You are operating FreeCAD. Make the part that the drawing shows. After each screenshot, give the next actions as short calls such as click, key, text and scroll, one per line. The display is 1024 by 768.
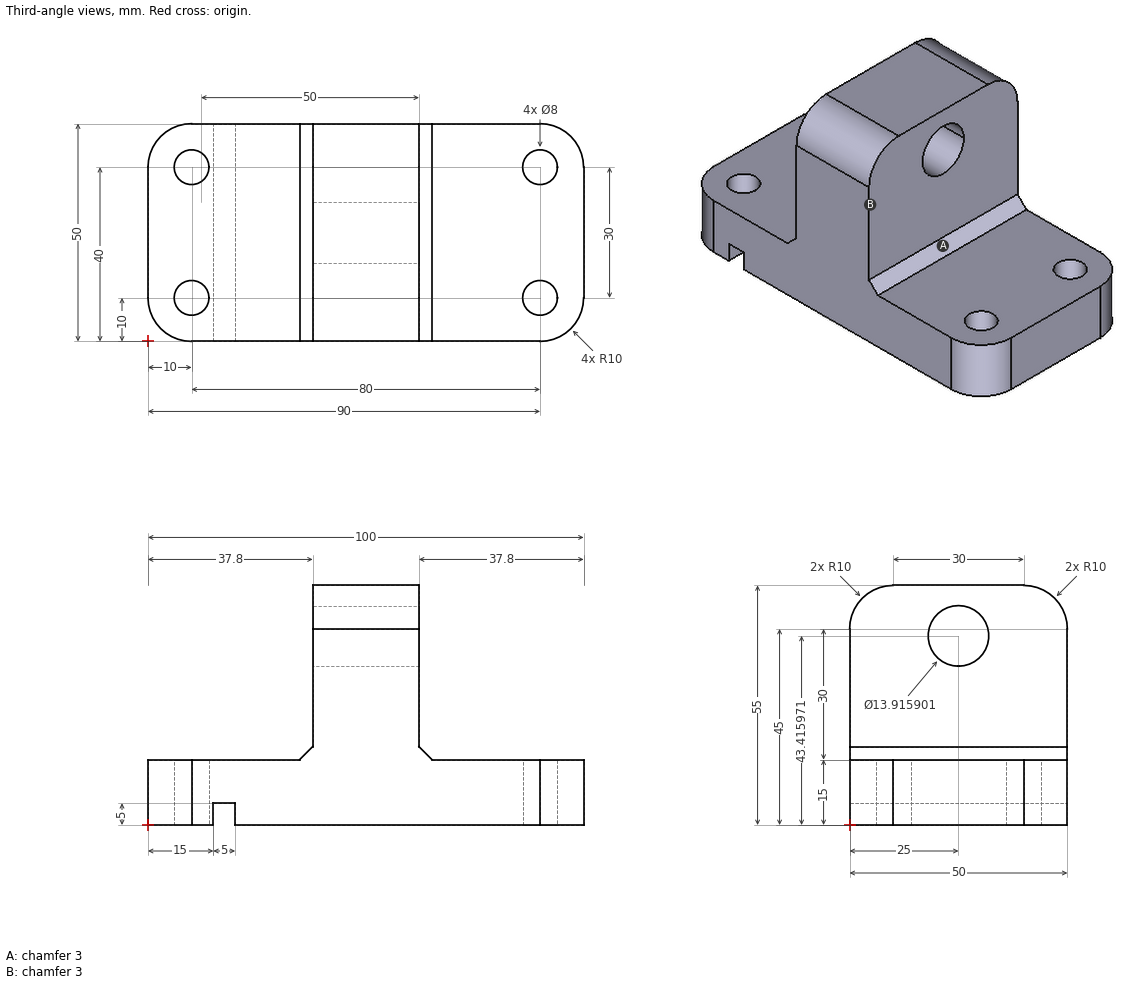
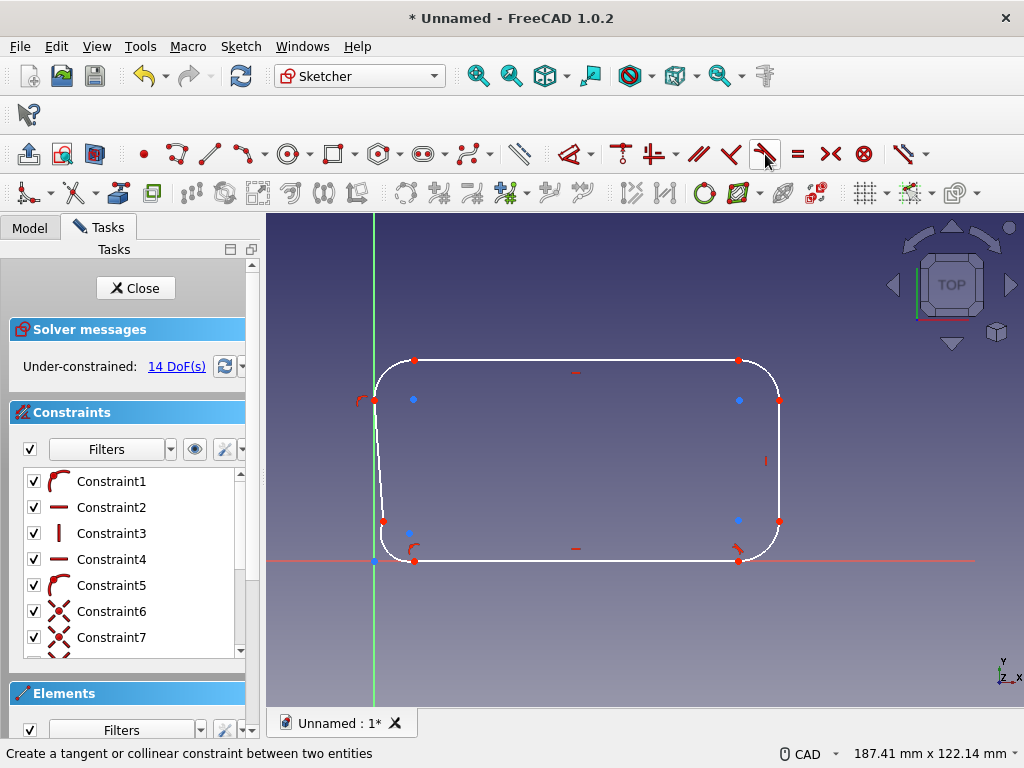
click(512, 561)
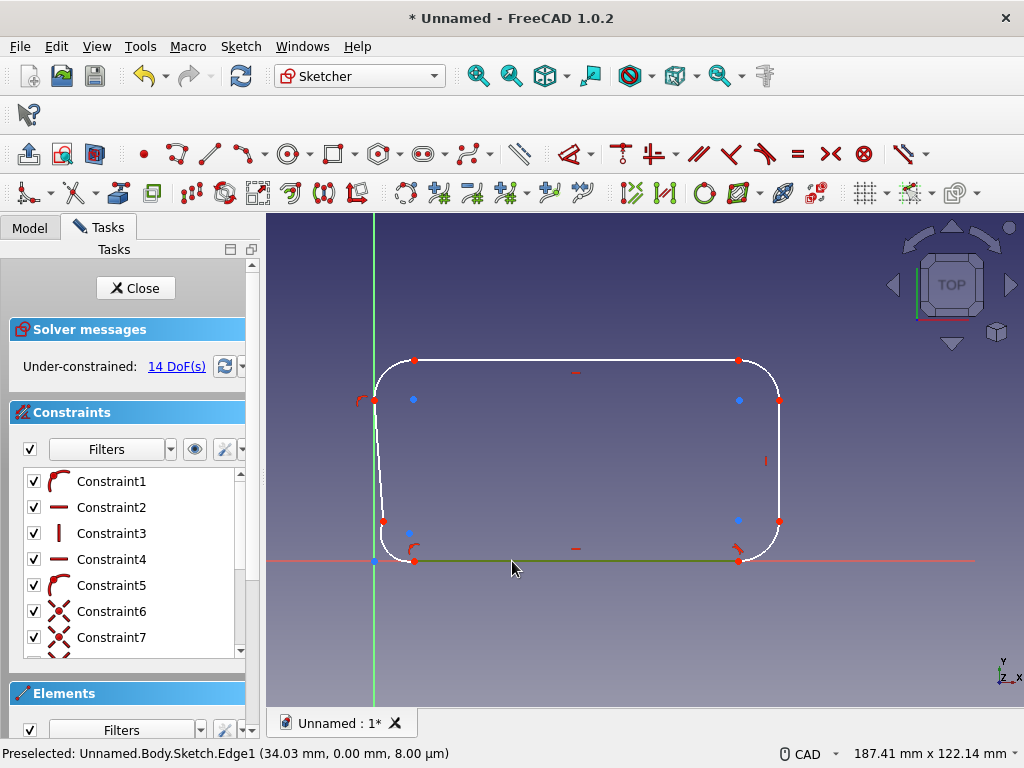
click(396, 558)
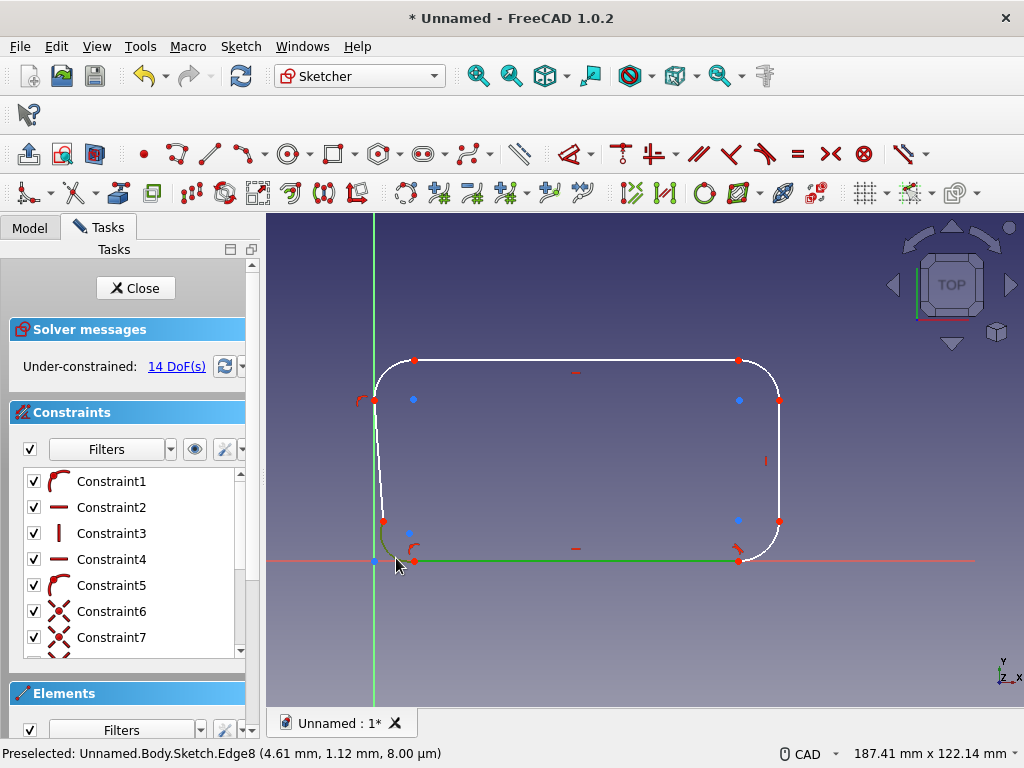
click(765, 154)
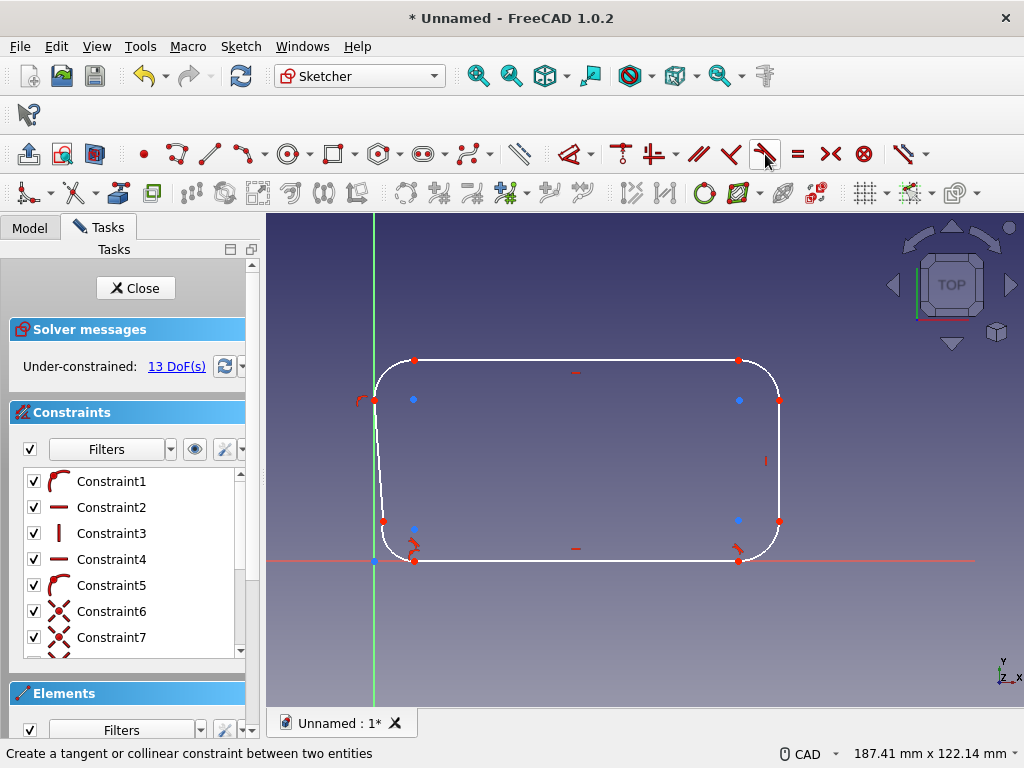
click(779, 485)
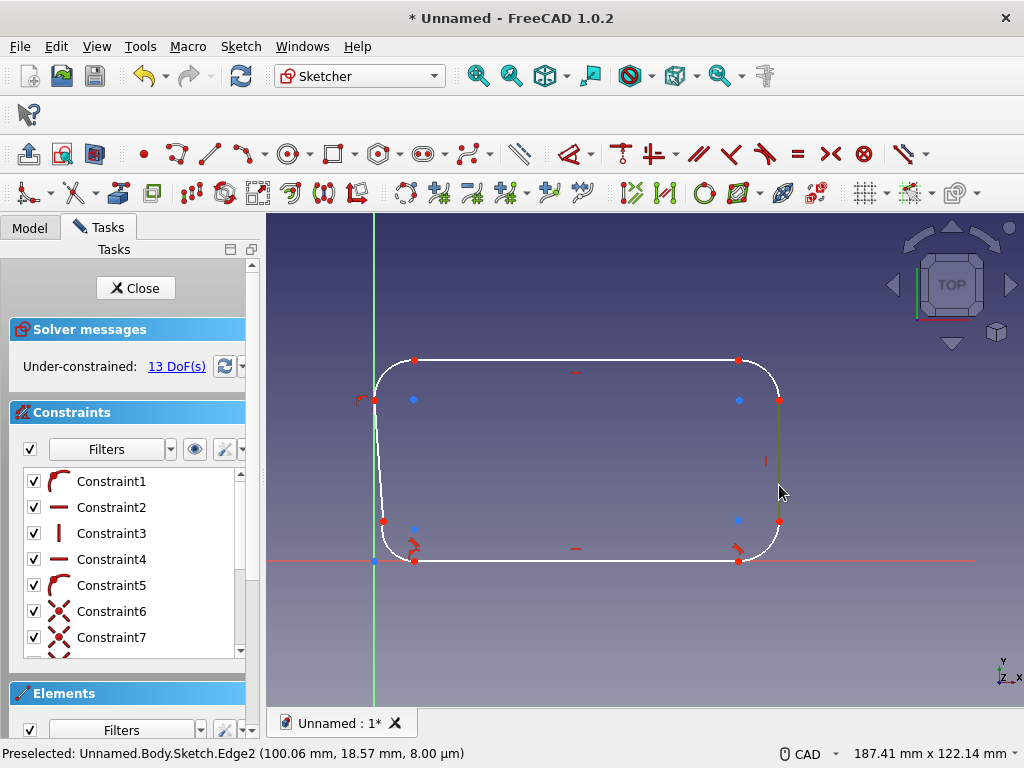
click(774, 539)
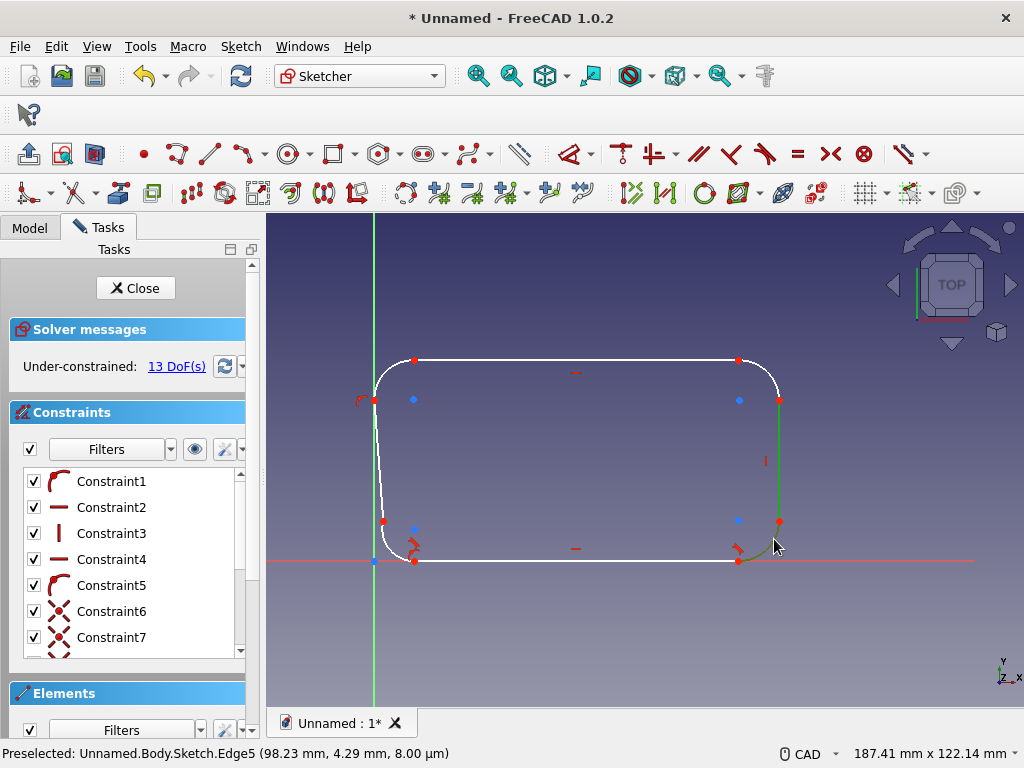
click(765, 154)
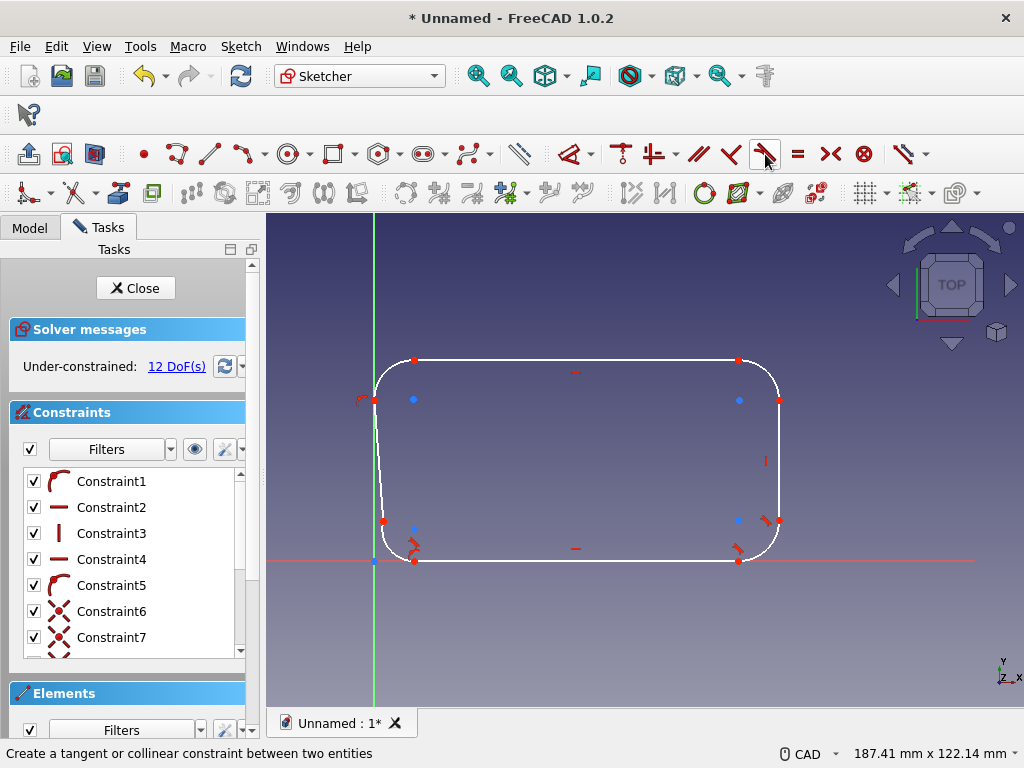
click(779, 484)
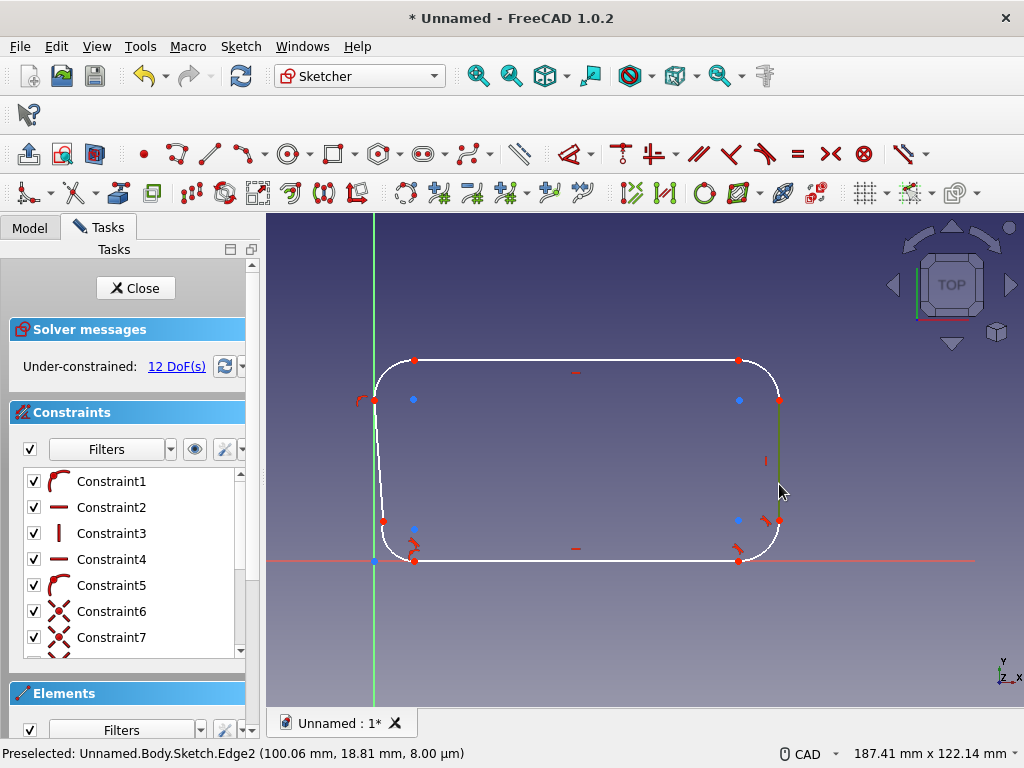
click(775, 382)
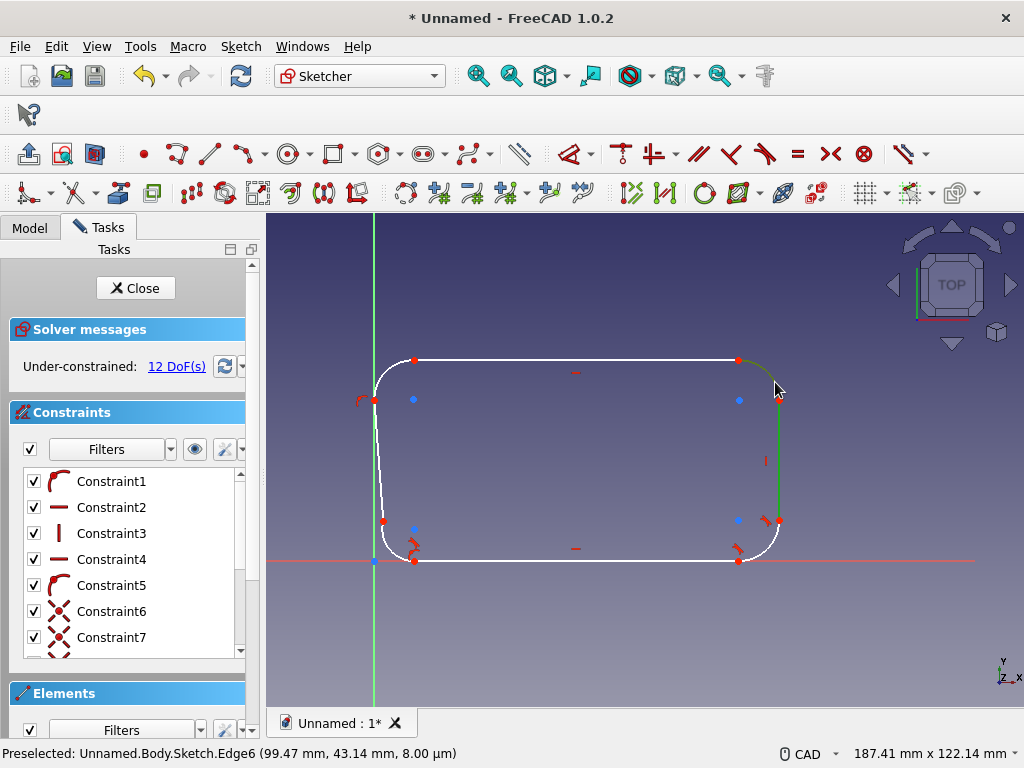
click(765, 154)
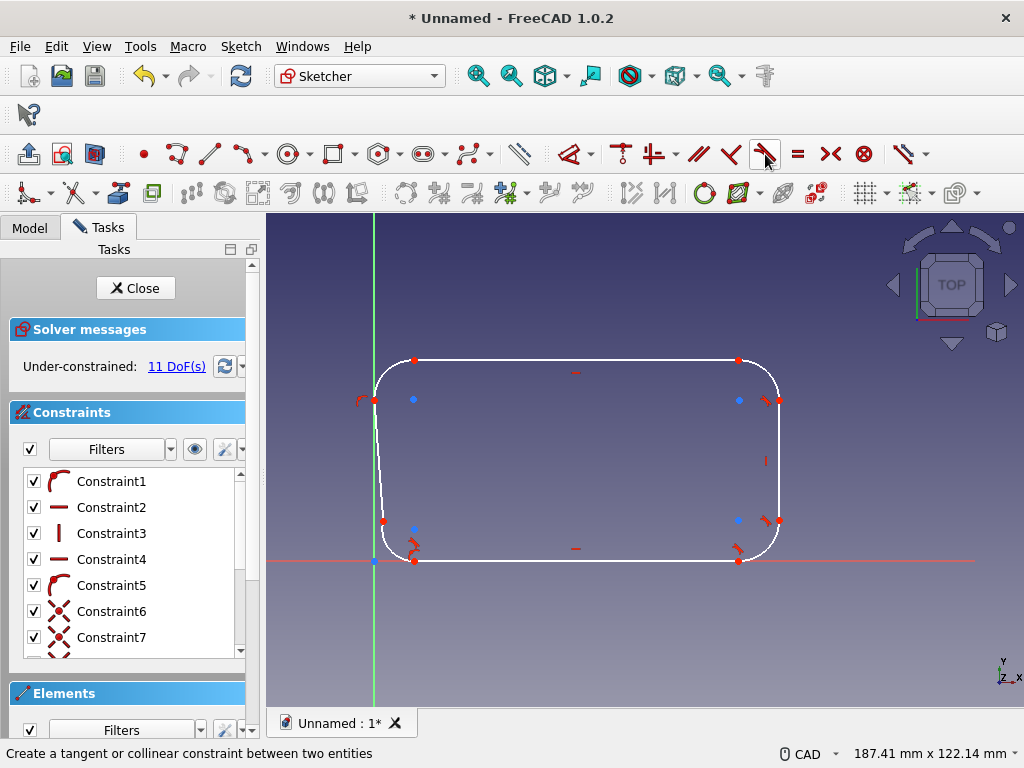
click(641, 360)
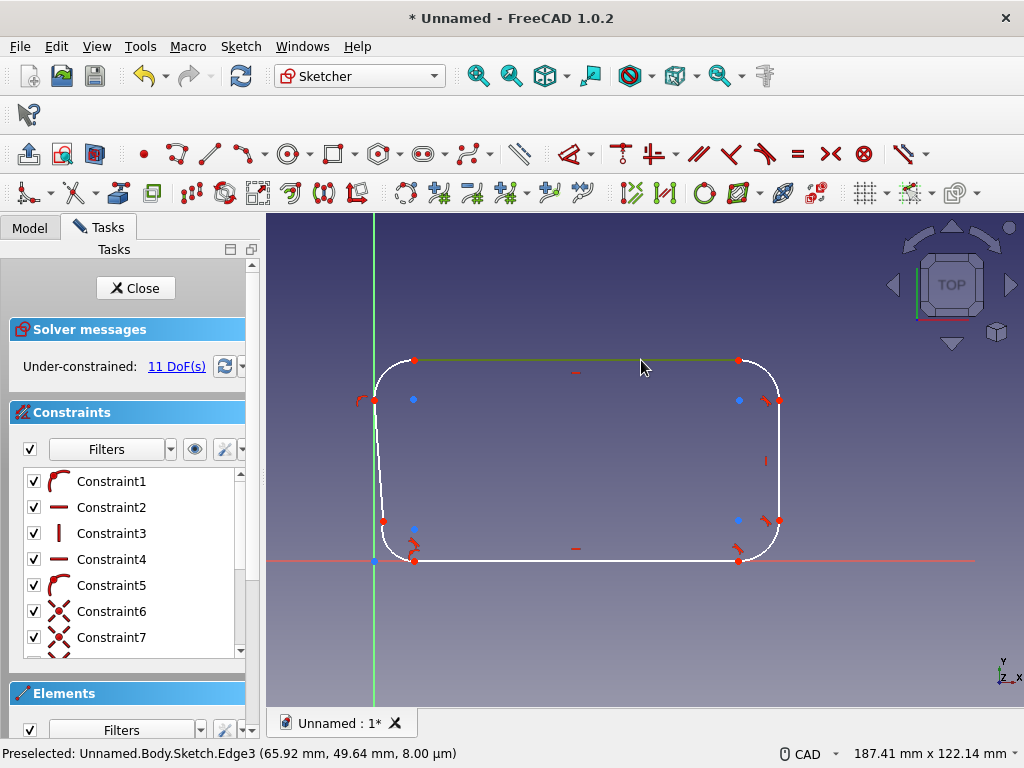
click(775, 382)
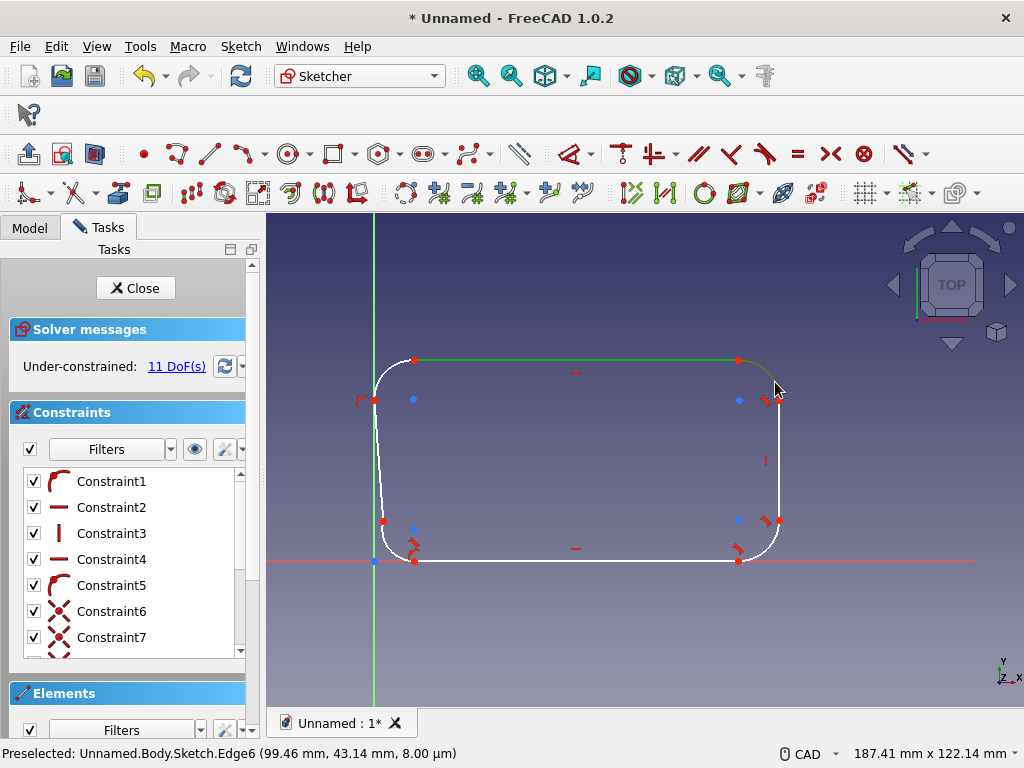
click(765, 154)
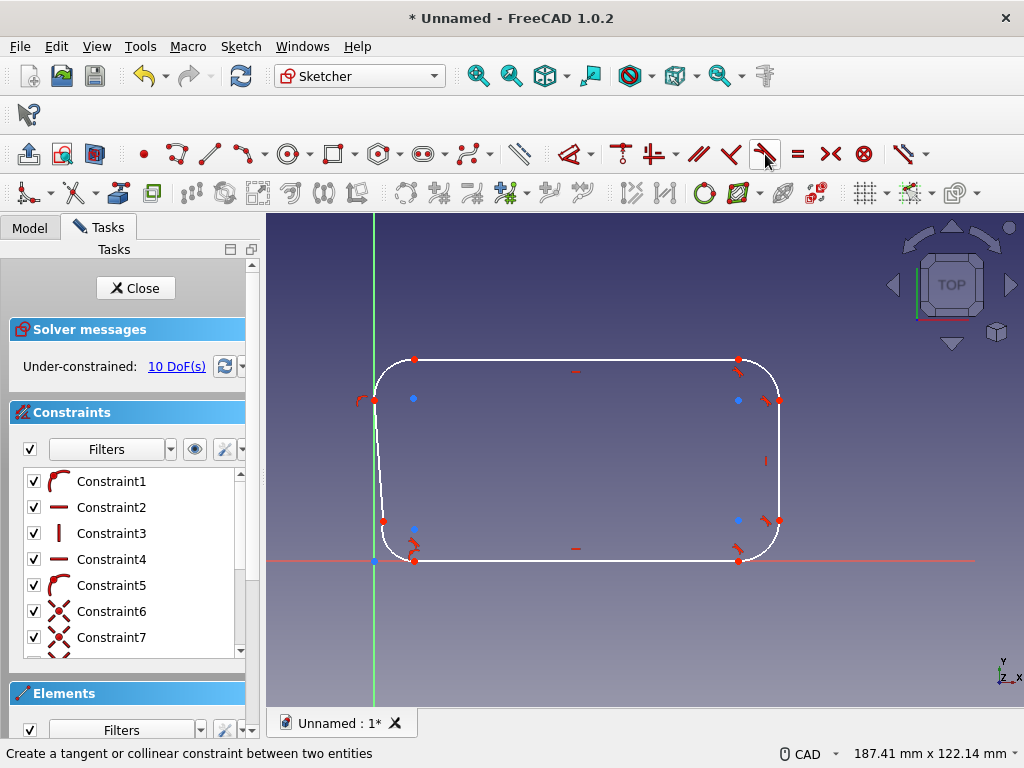
click(641, 360)